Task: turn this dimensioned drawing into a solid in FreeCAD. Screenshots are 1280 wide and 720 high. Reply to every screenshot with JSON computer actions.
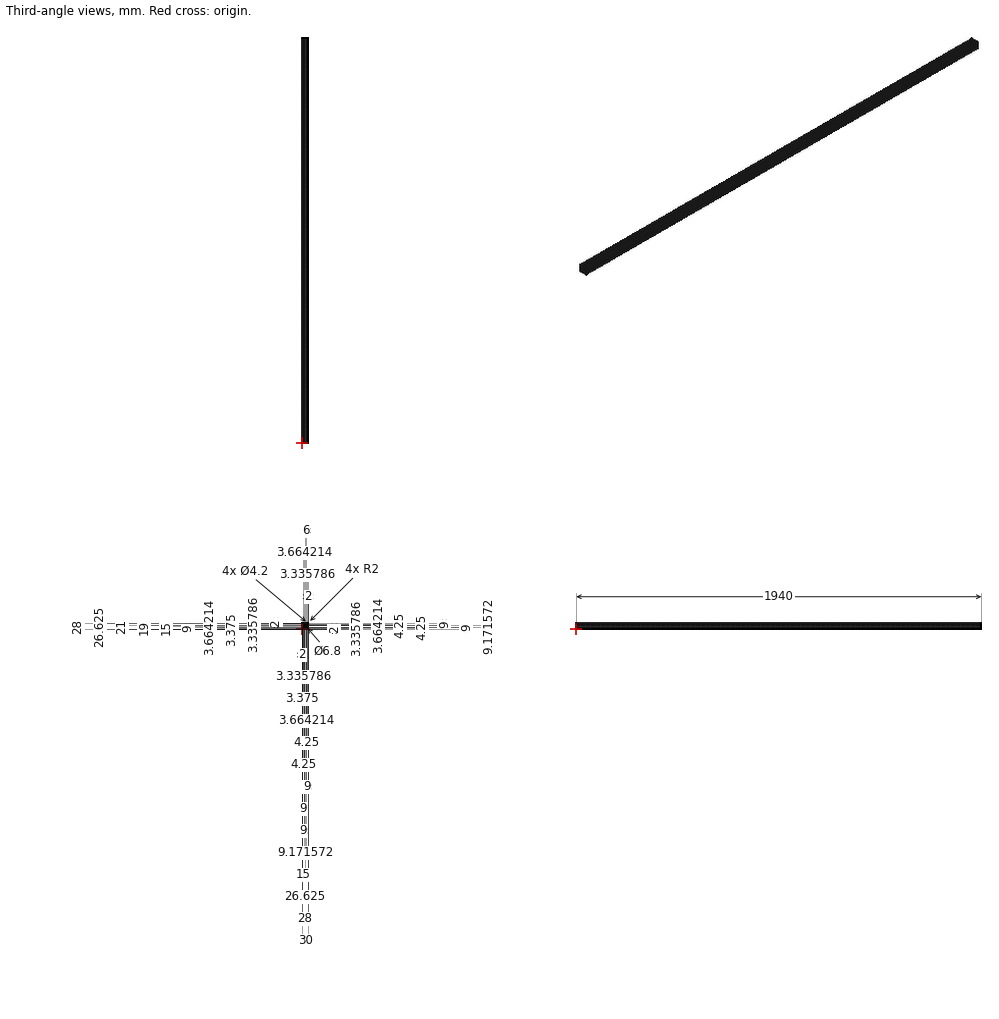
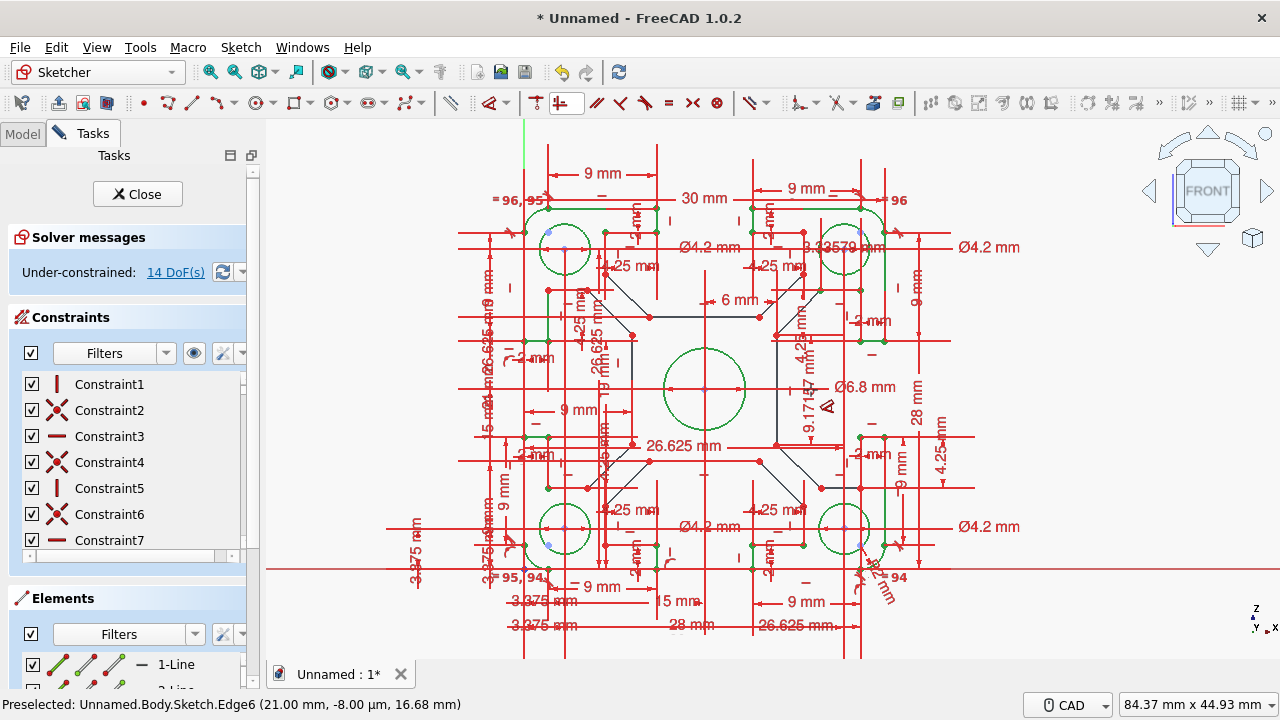
{"action": "left_click", "coordinate": [833, 488]}
{"action": "left_click", "coordinate": [850, 522]}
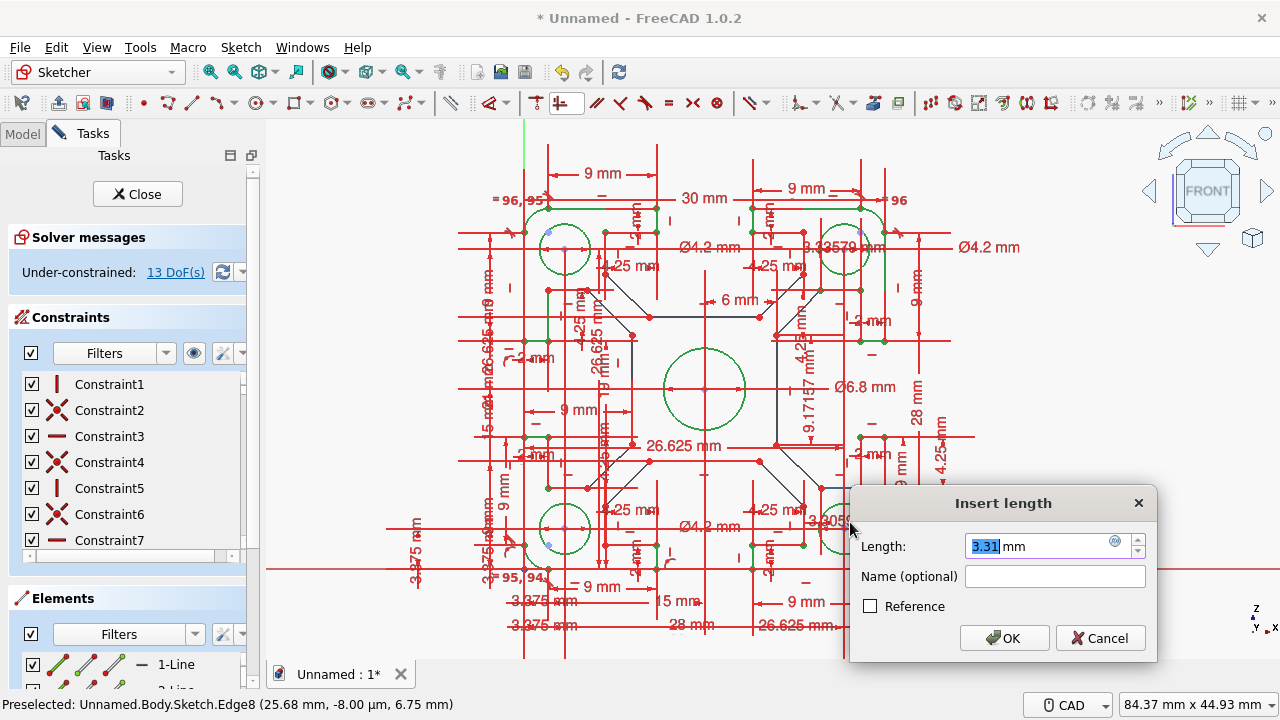
{"action": "type", "text": "3.335786"}
{"action": "key", "text": "Return"}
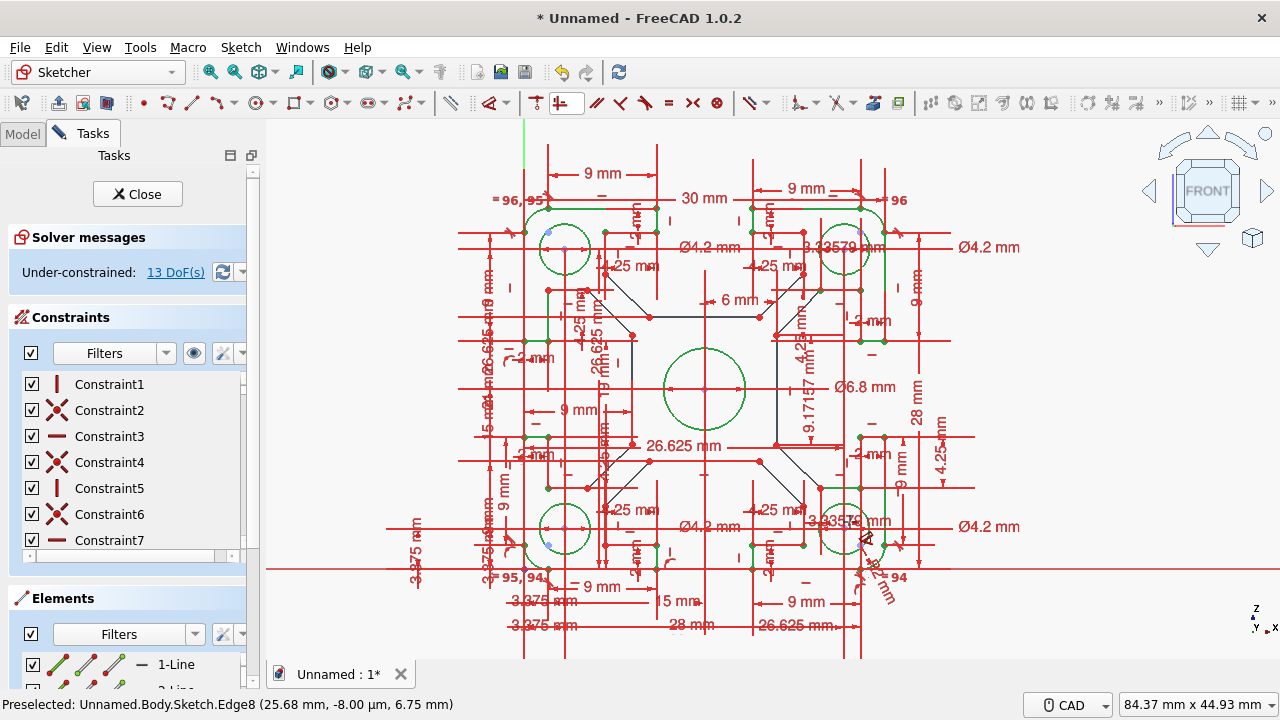
{"action": "left_click", "coordinate": [804, 534]}
{"action": "left_click", "coordinate": [722, 535]}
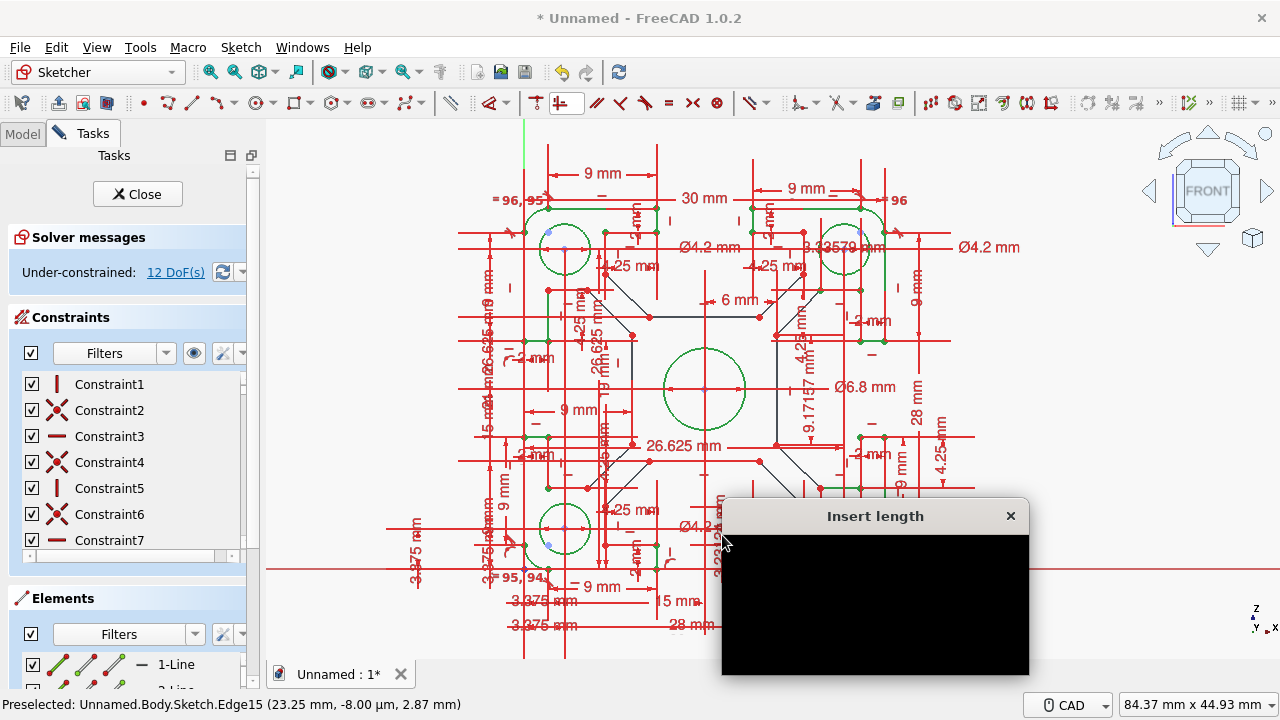
{"action": "type", "text": "3.335786"}
{"action": "key", "text": "Return"}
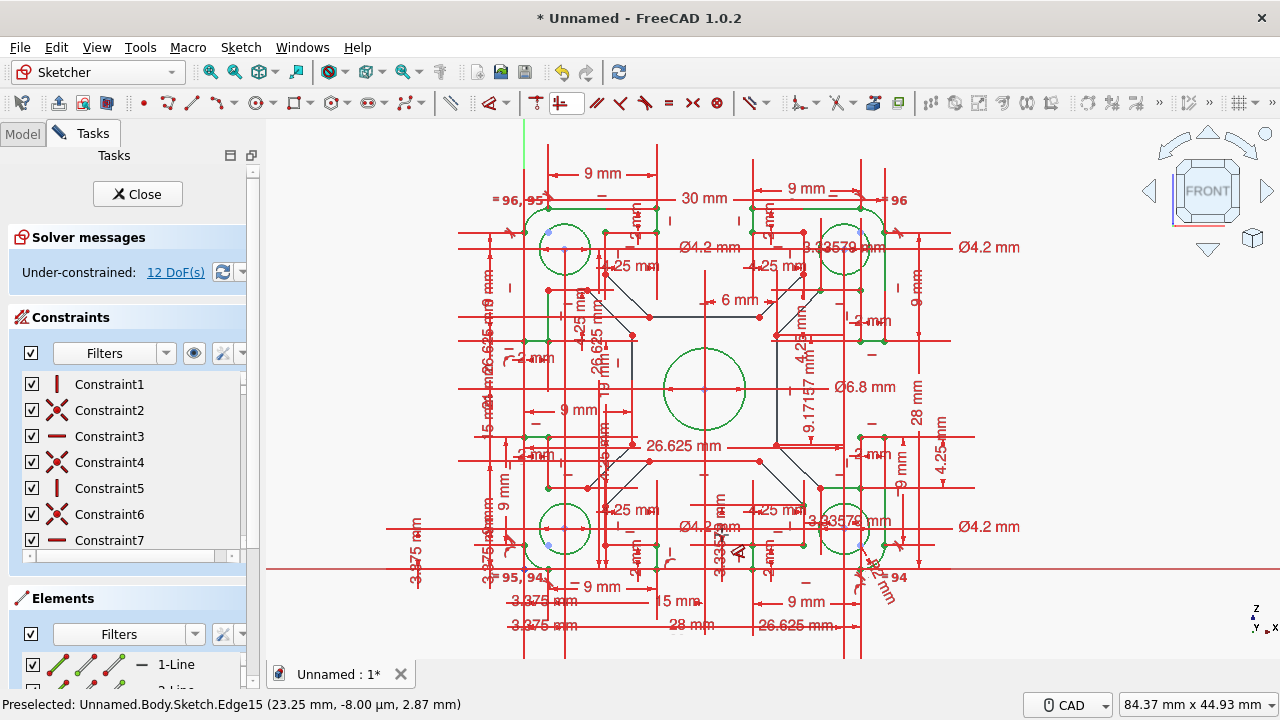
{"action": "left_click", "coordinate": [726, 461]}
{"action": "left_click", "coordinate": [705, 495]}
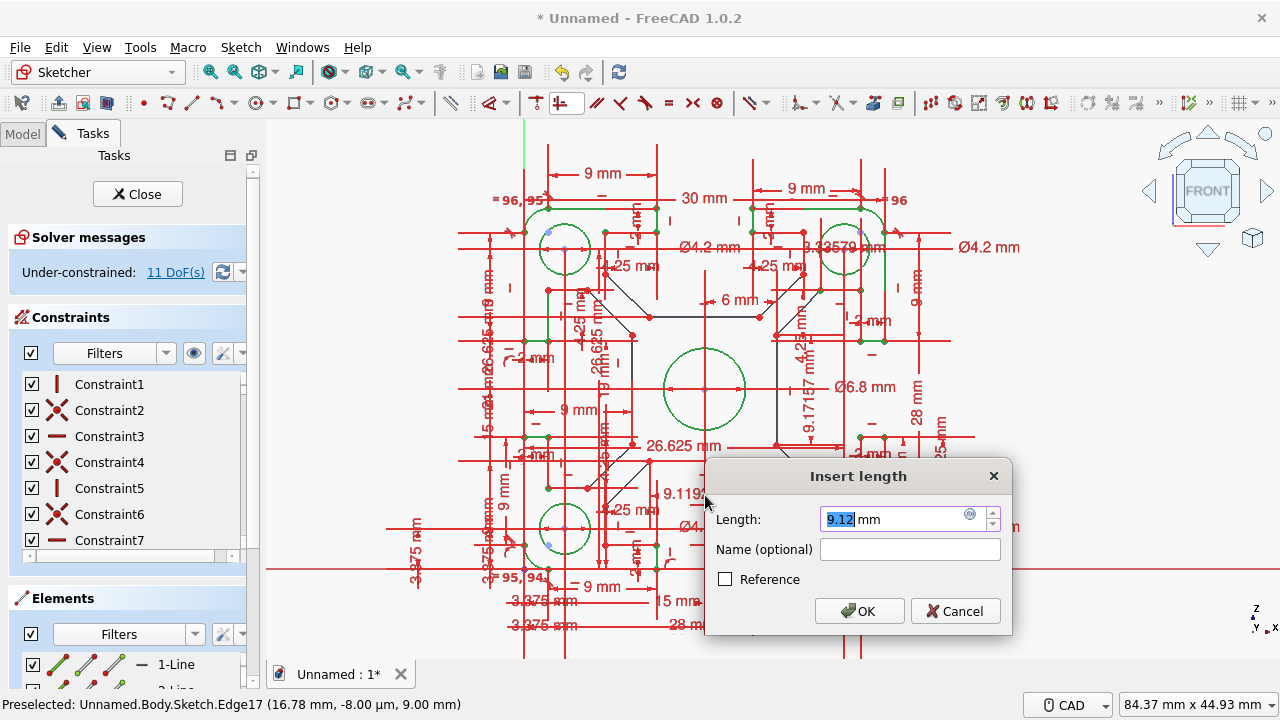
{"action": "type", "text": "9.171572"}
{"action": "key", "text": "Return"}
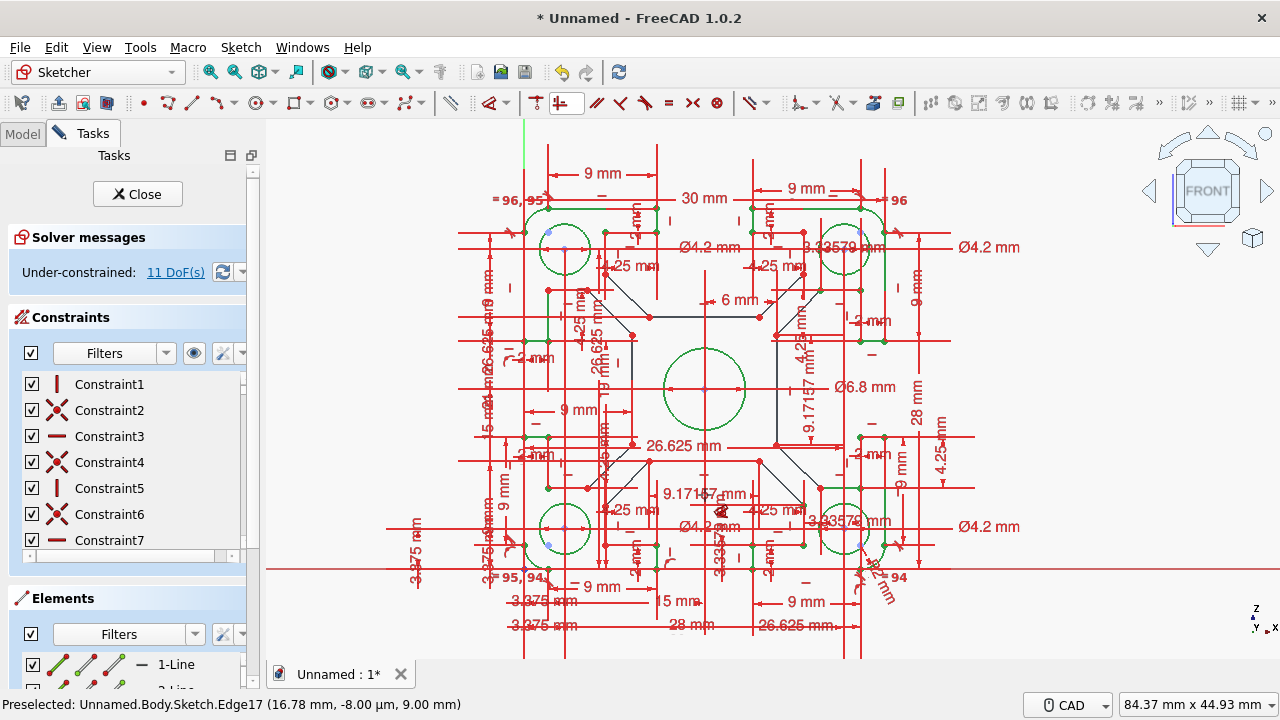
{"action": "left_click", "coordinate": [605, 518]}
{"action": "left_click", "coordinate": [571, 535]}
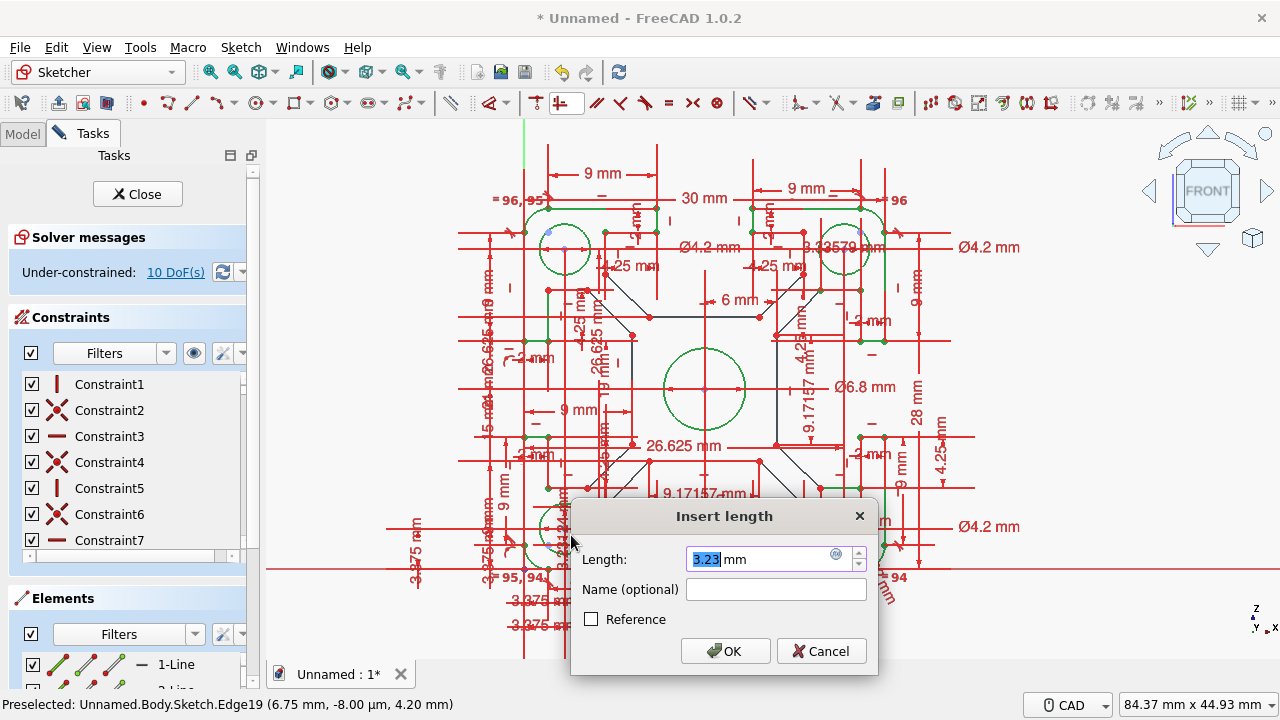
{"action": "type", "text": "3.335786"}
{"action": "key", "text": "Return"}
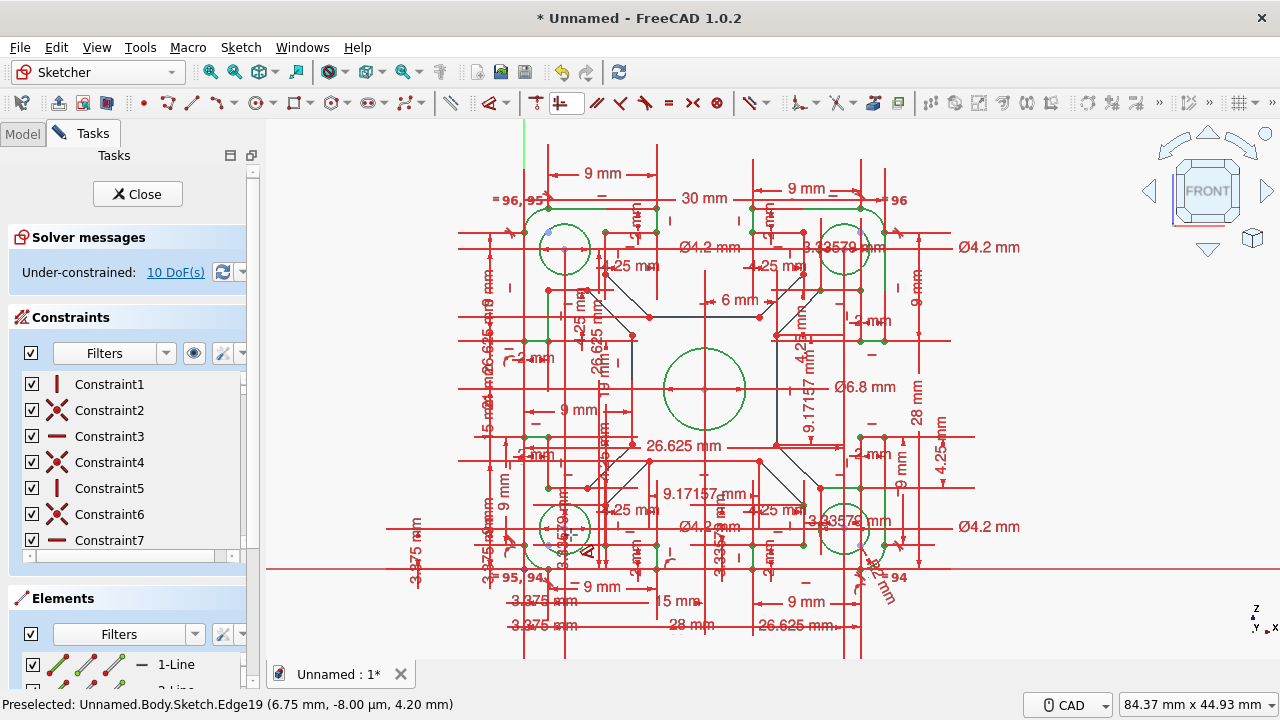
{"action": "left_click", "coordinate": [560, 488]}
{"action": "left_click", "coordinate": [568, 522]}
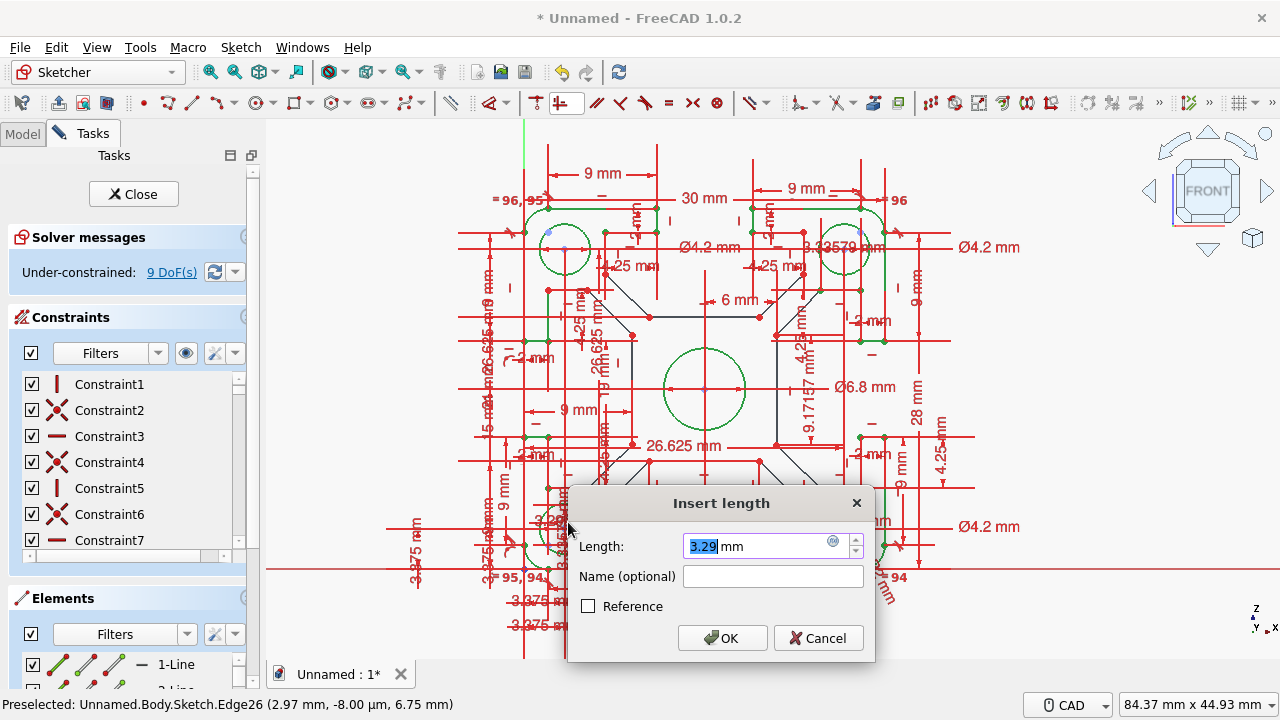
{"action": "type", "text": "3.335786"}
{"action": "key", "text": "Return"}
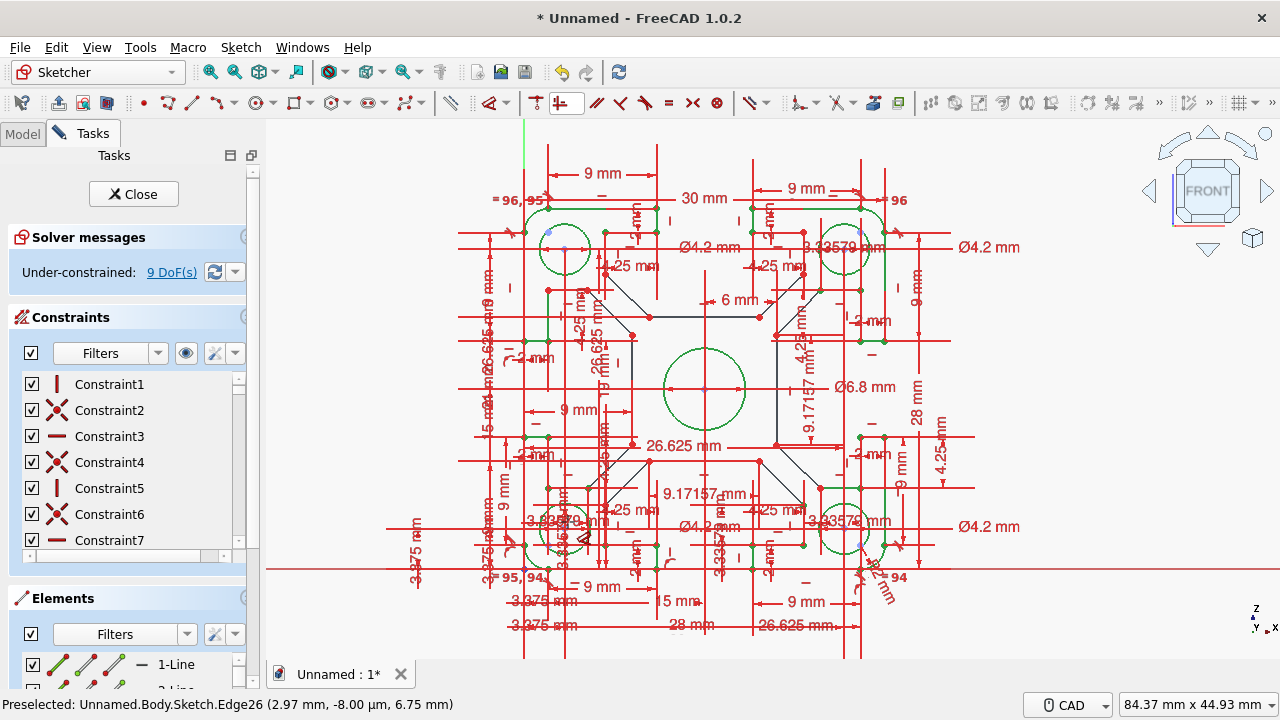
{"action": "left_click", "coordinate": [632, 412]}
{"action": "left_click", "coordinate": [690, 390]}